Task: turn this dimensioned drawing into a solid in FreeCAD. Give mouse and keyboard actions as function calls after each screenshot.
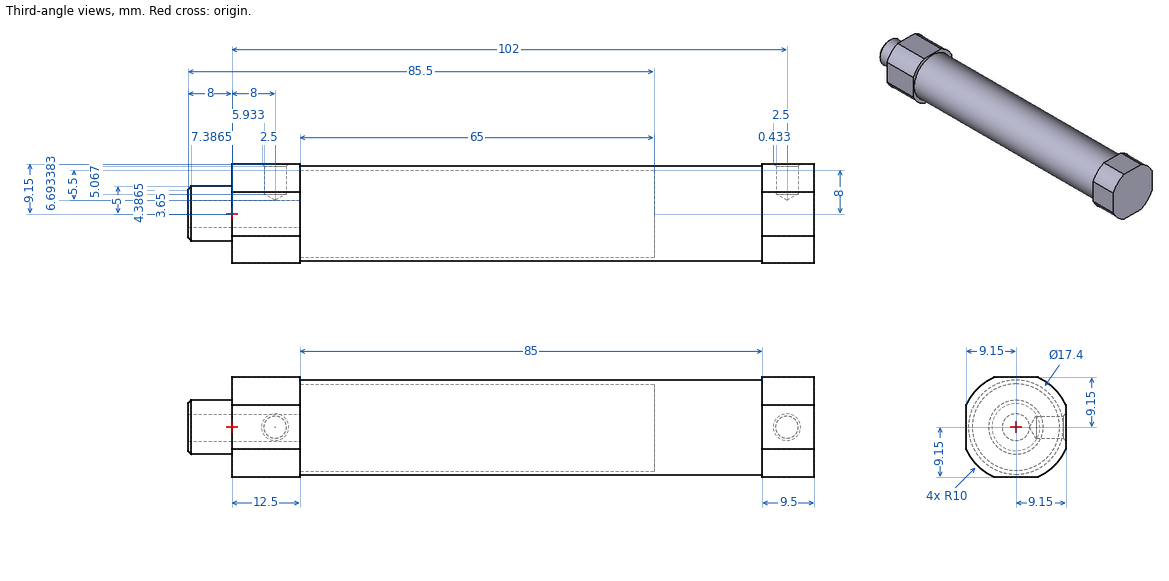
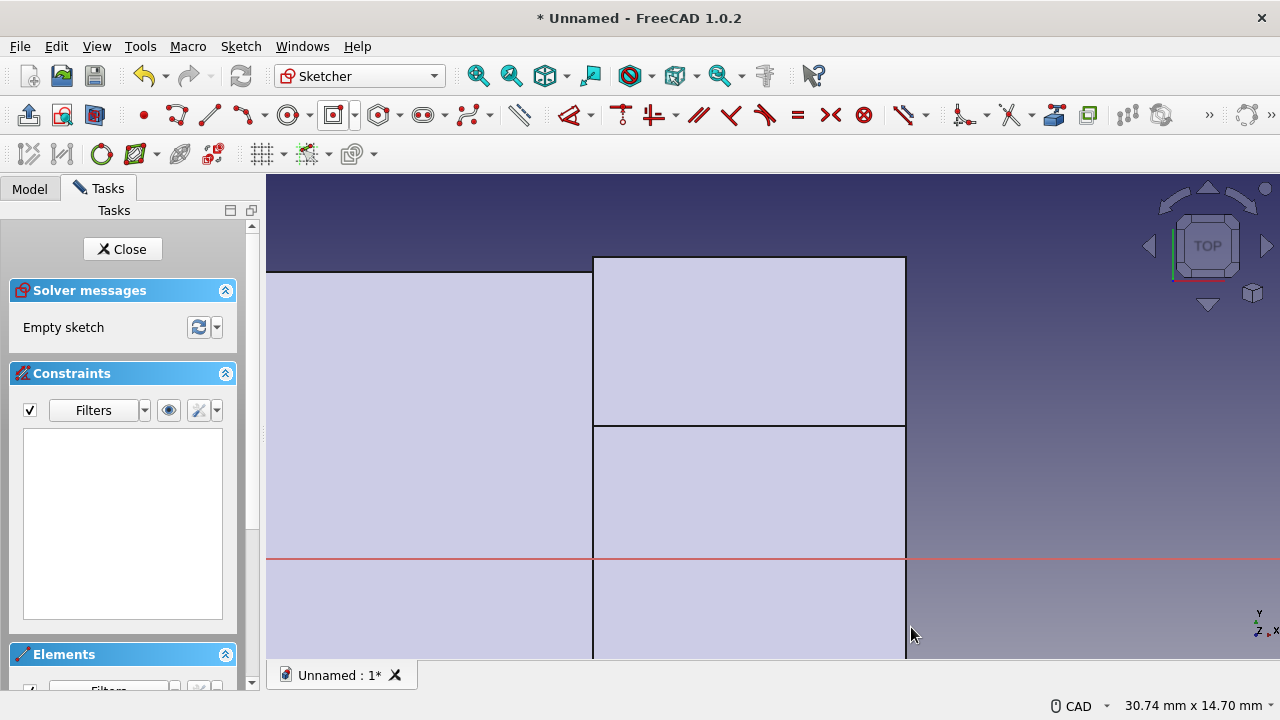
click(177, 116)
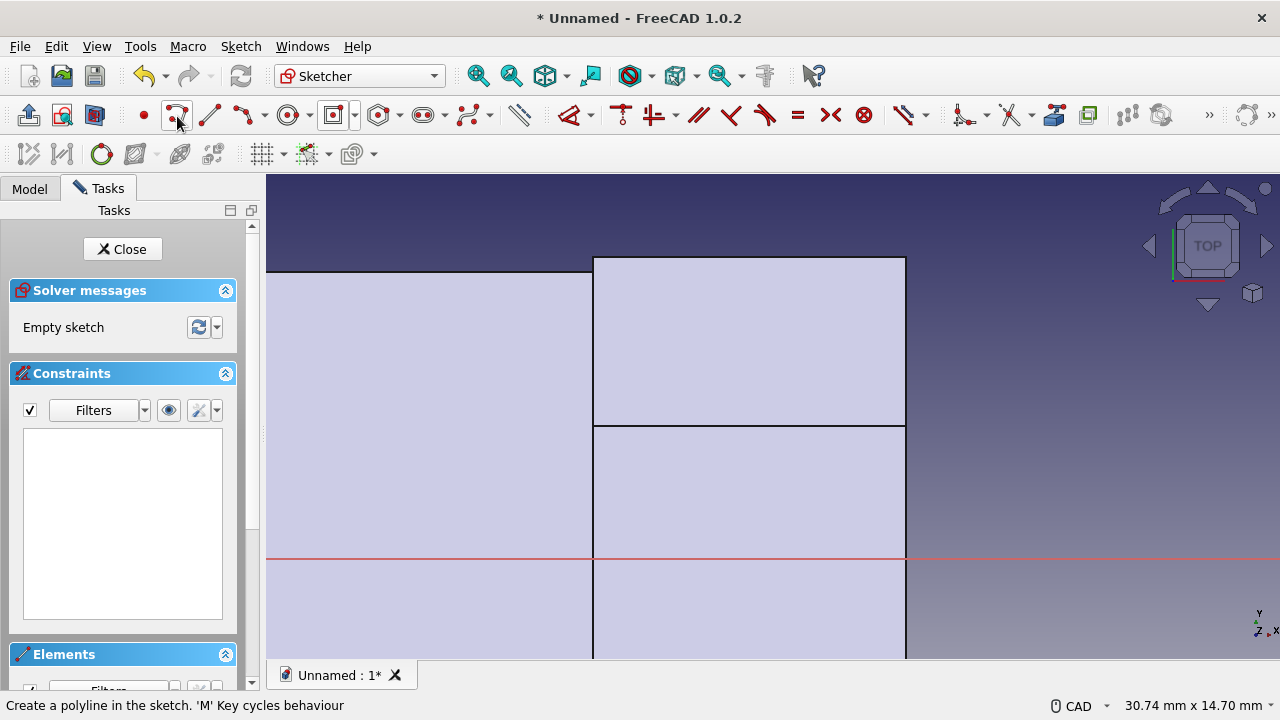
click(659, 257)
click(673, 271)
click(673, 438)
click(741, 478)
click(741, 257)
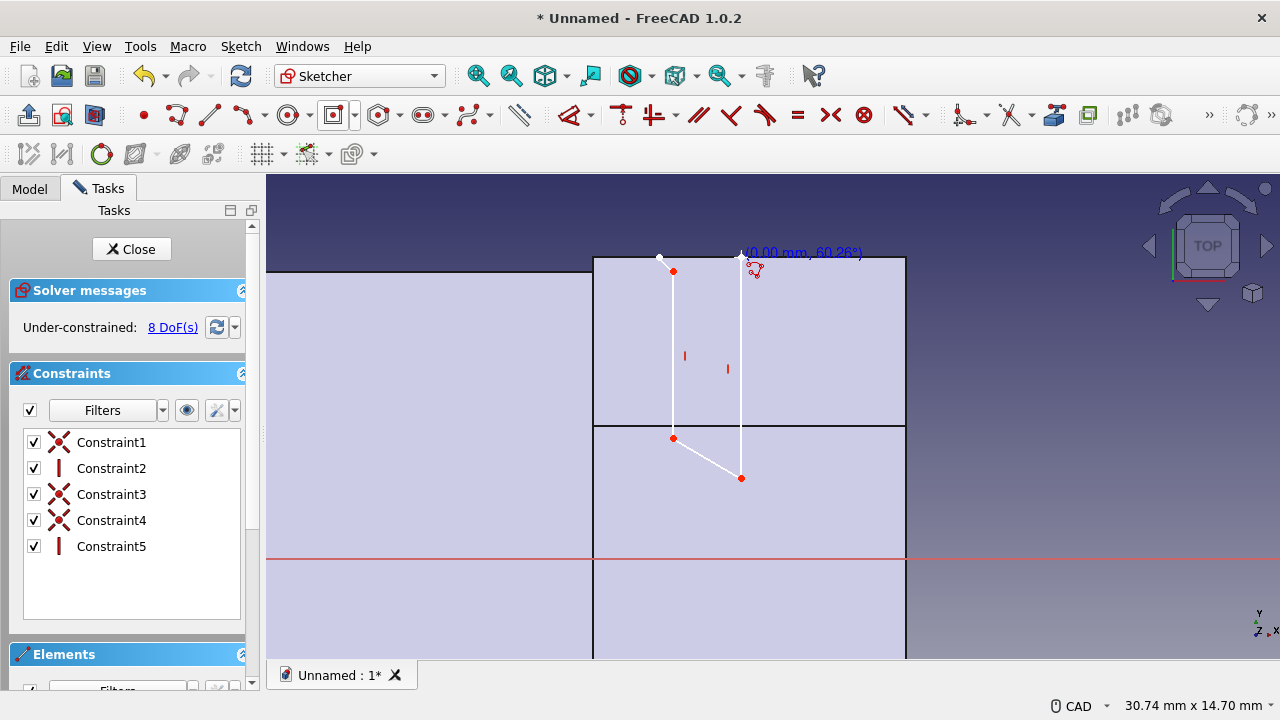
scroll(659, 257, up, 3)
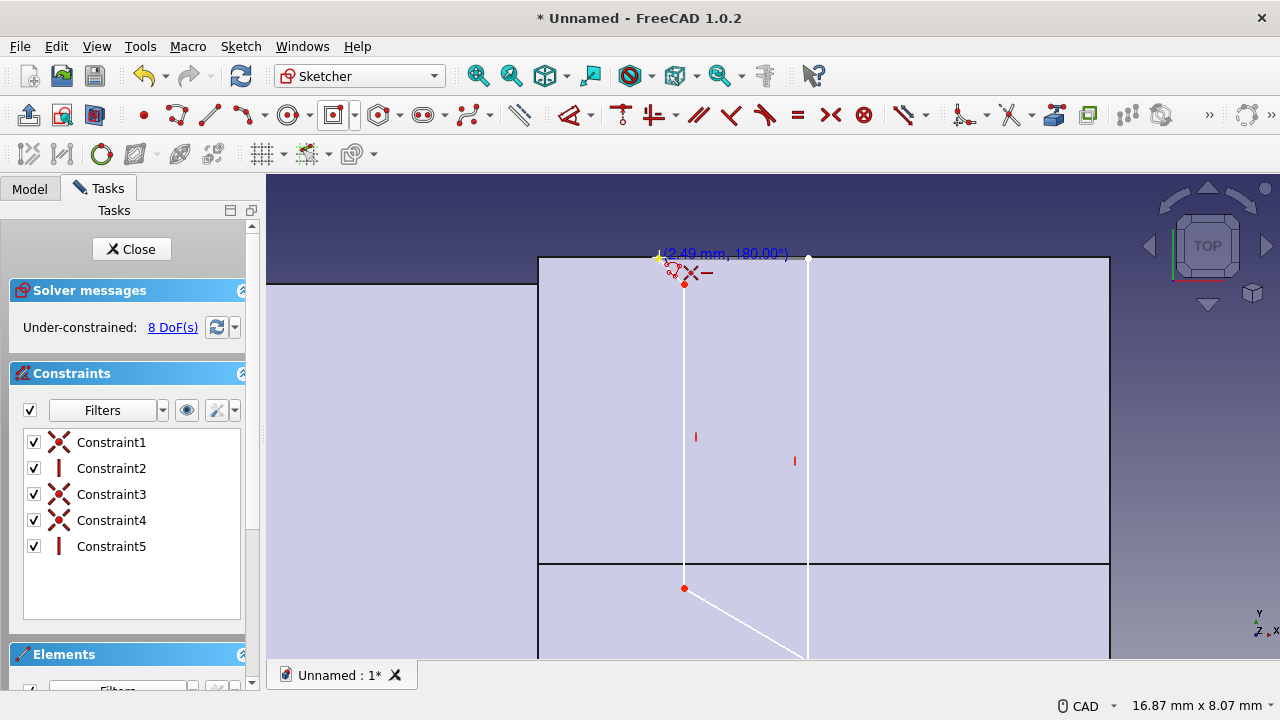
click(659, 259)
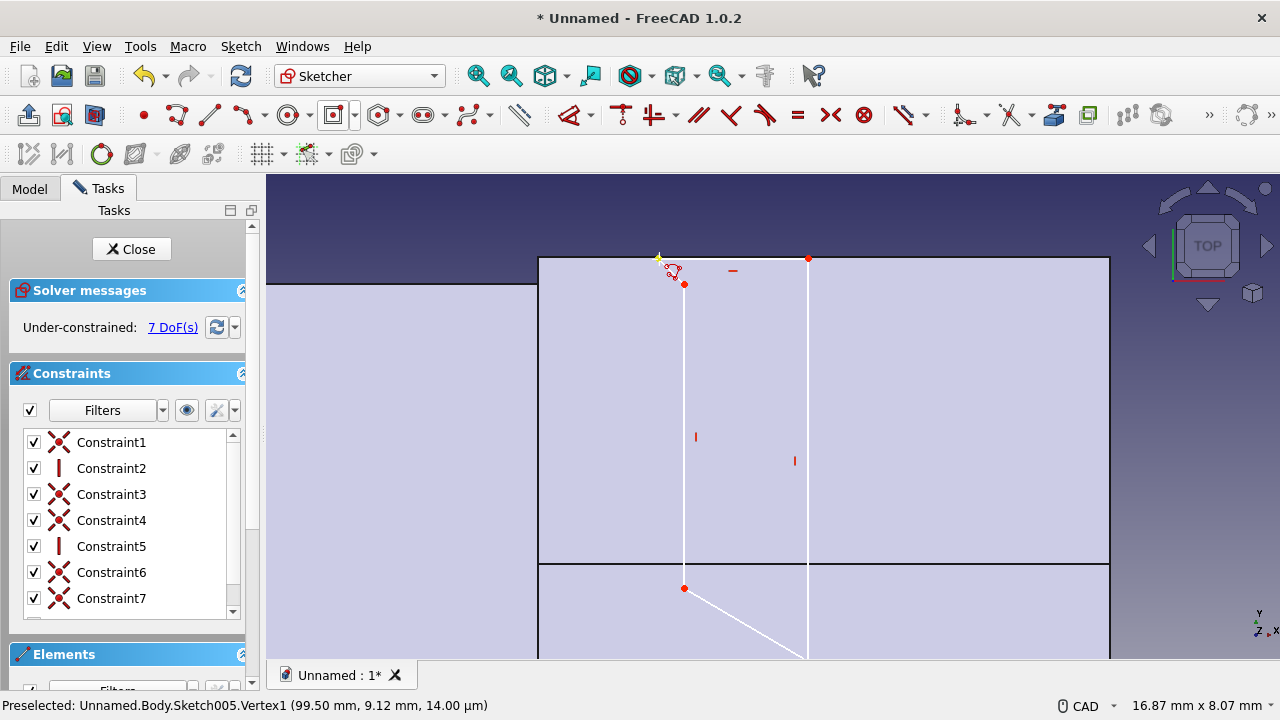
click(210, 116)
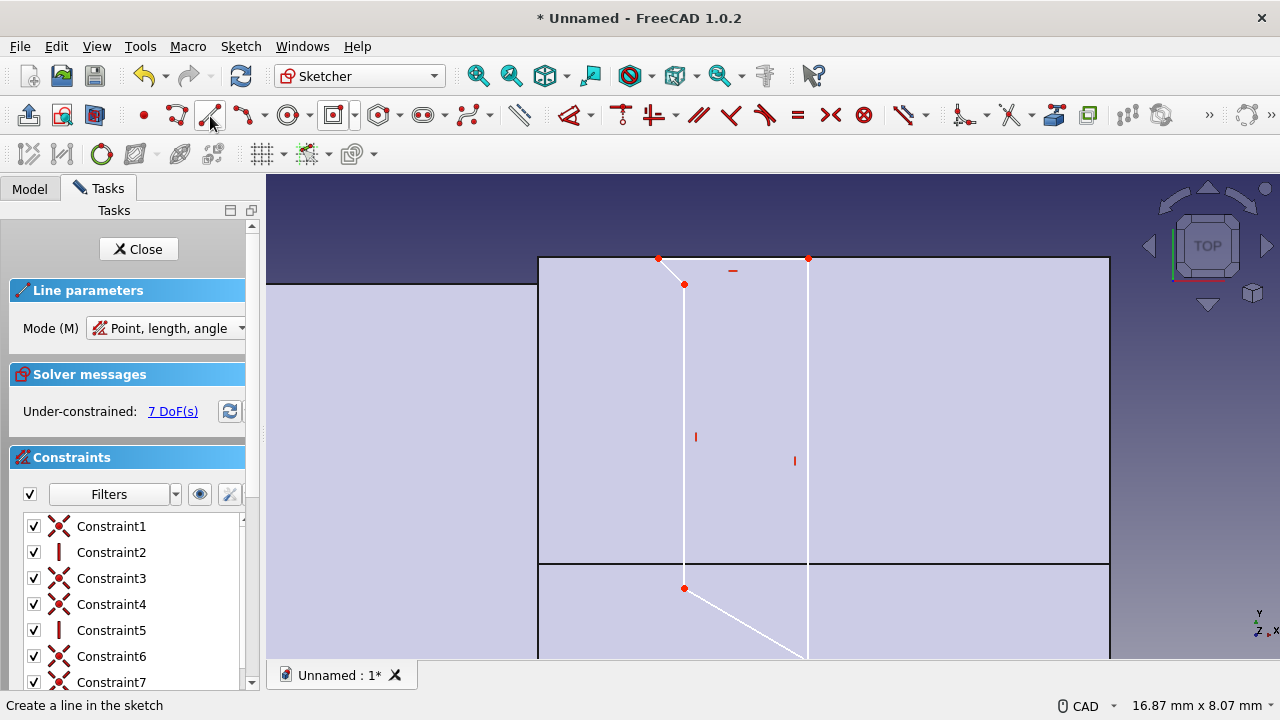
scroll(669, 268, down, 3)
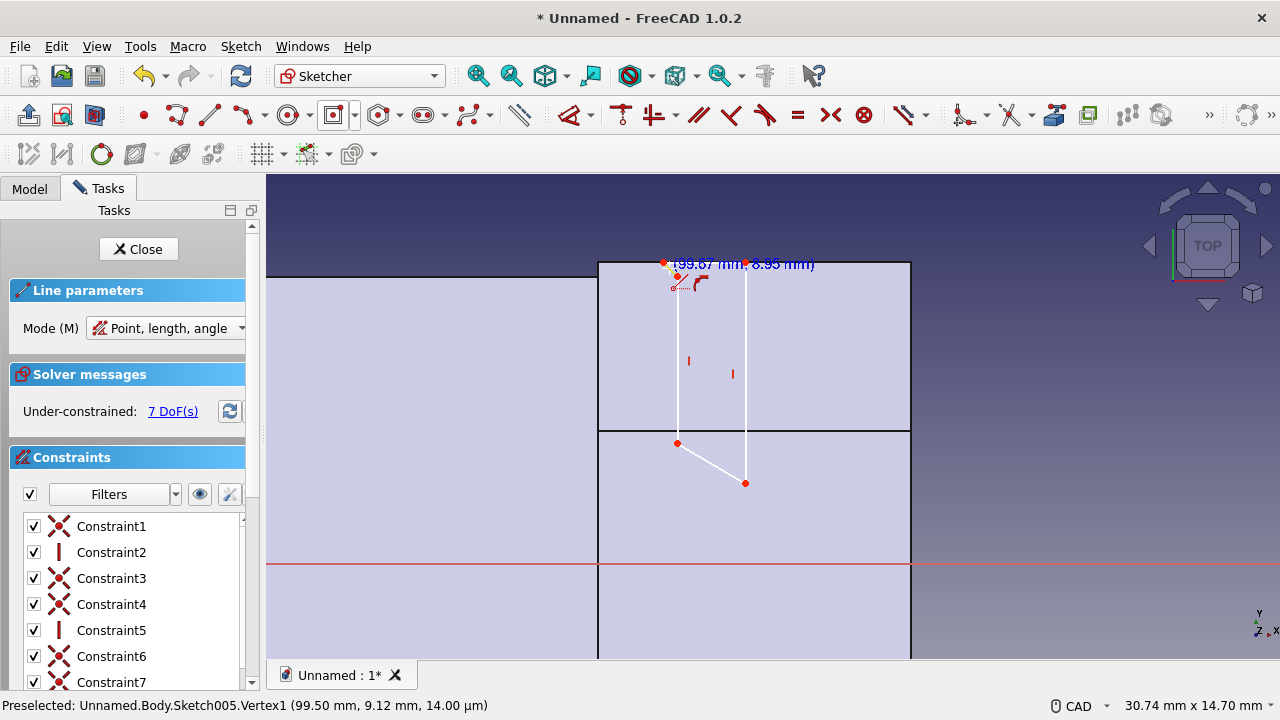
click(746, 505)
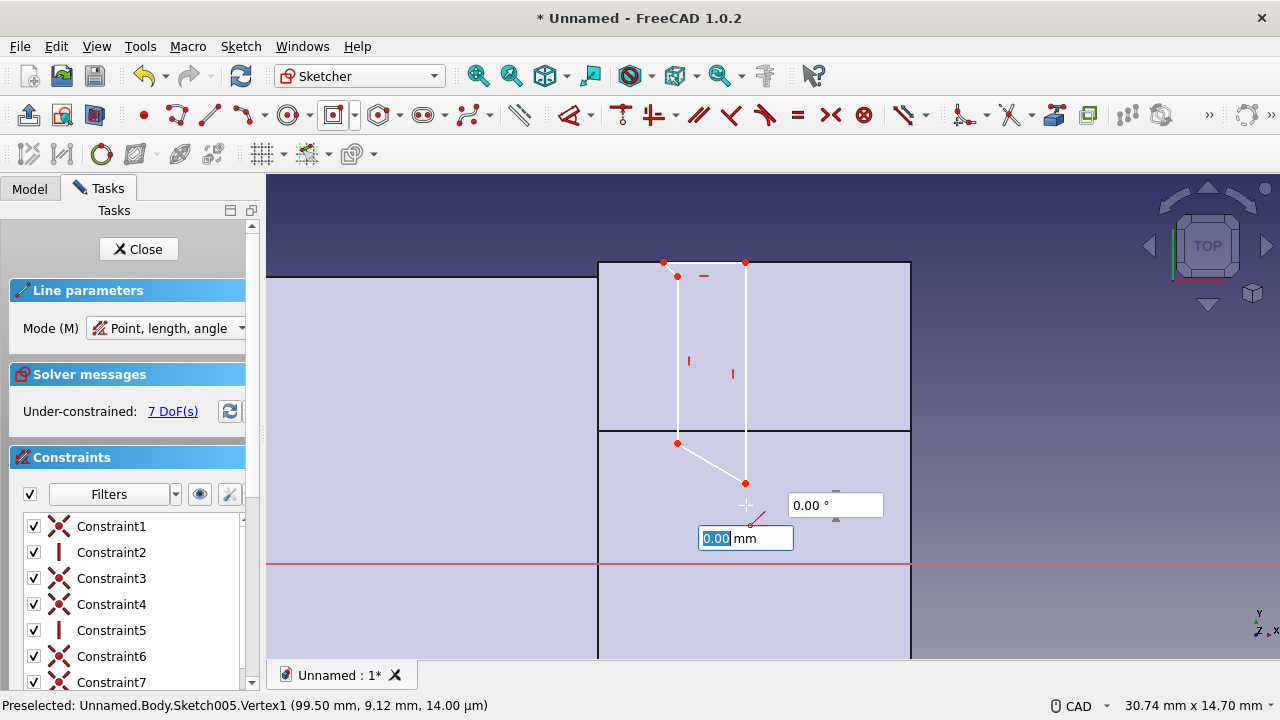
scroll(746, 571, up, 4)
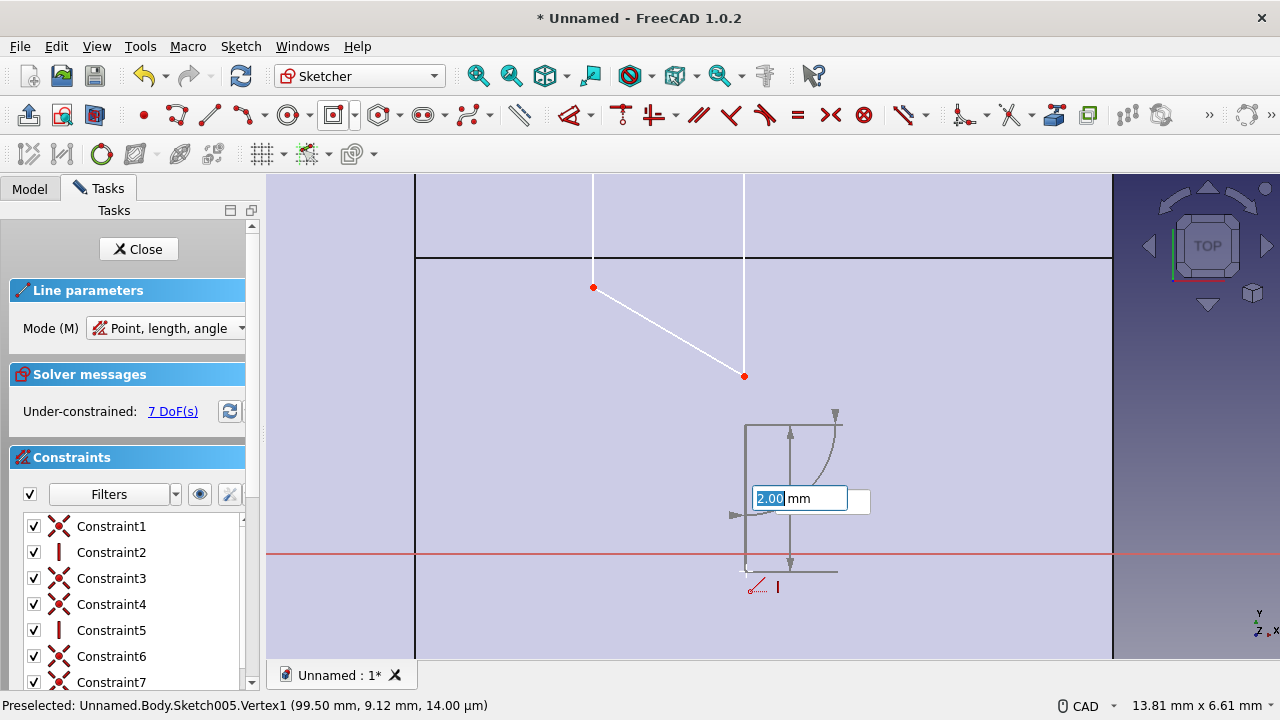
click(745, 570)
key(Escape)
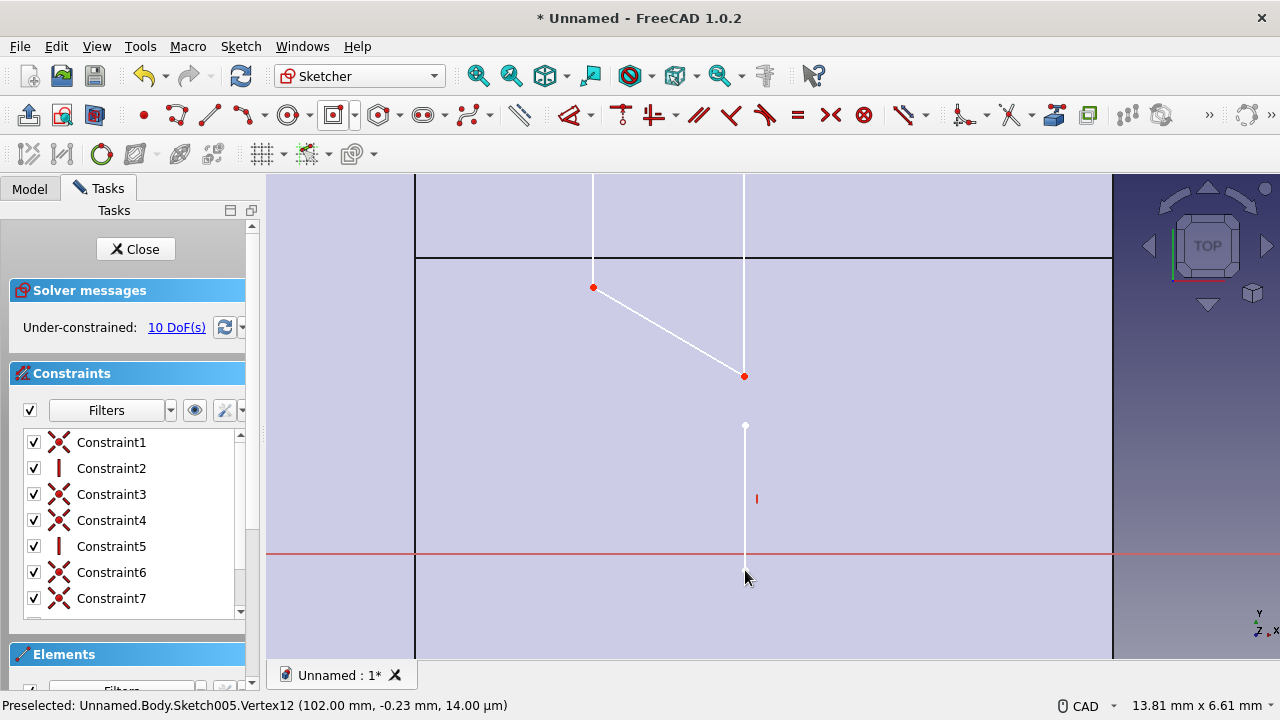
click(745, 469)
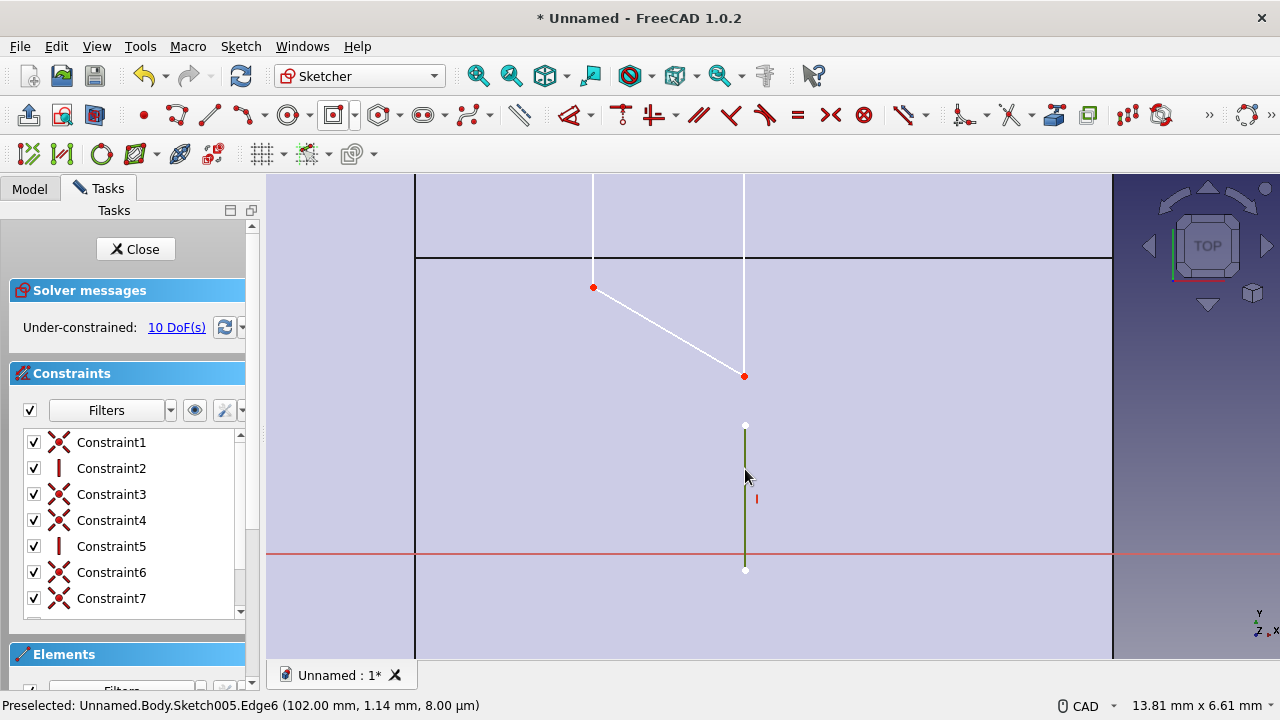
click(520, 116)